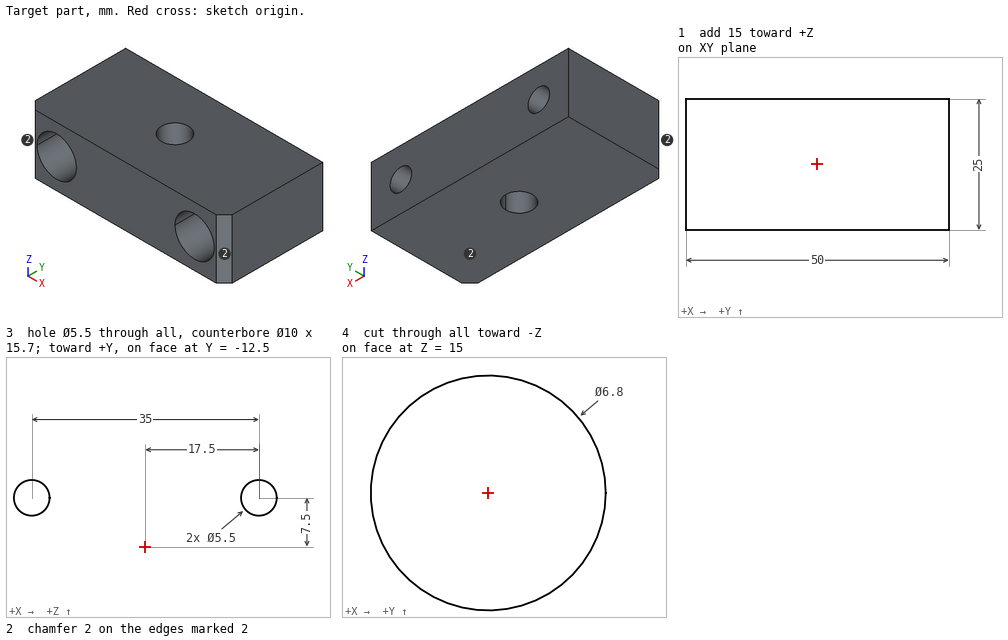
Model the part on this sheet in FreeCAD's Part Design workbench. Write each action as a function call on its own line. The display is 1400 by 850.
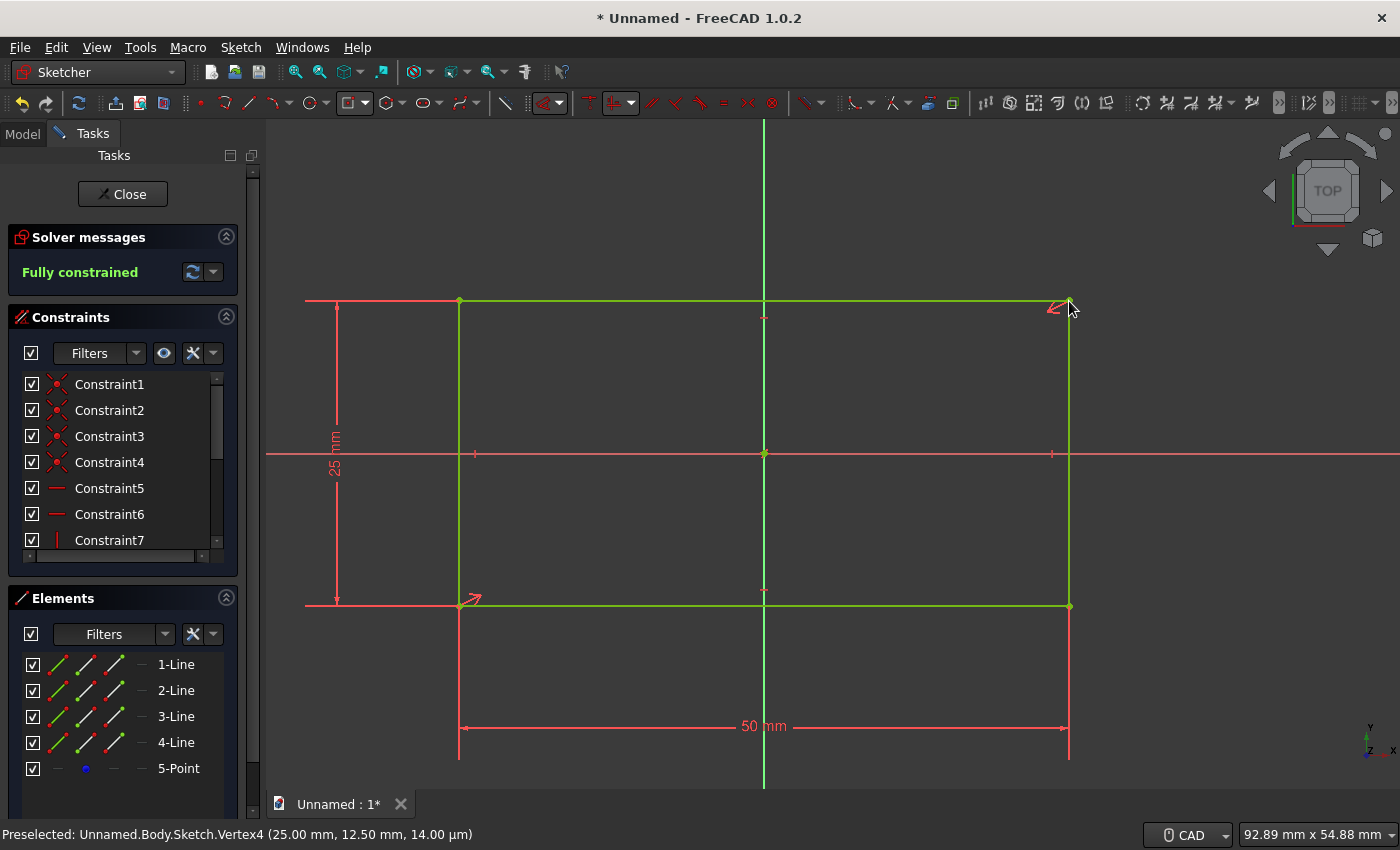
click(123, 194)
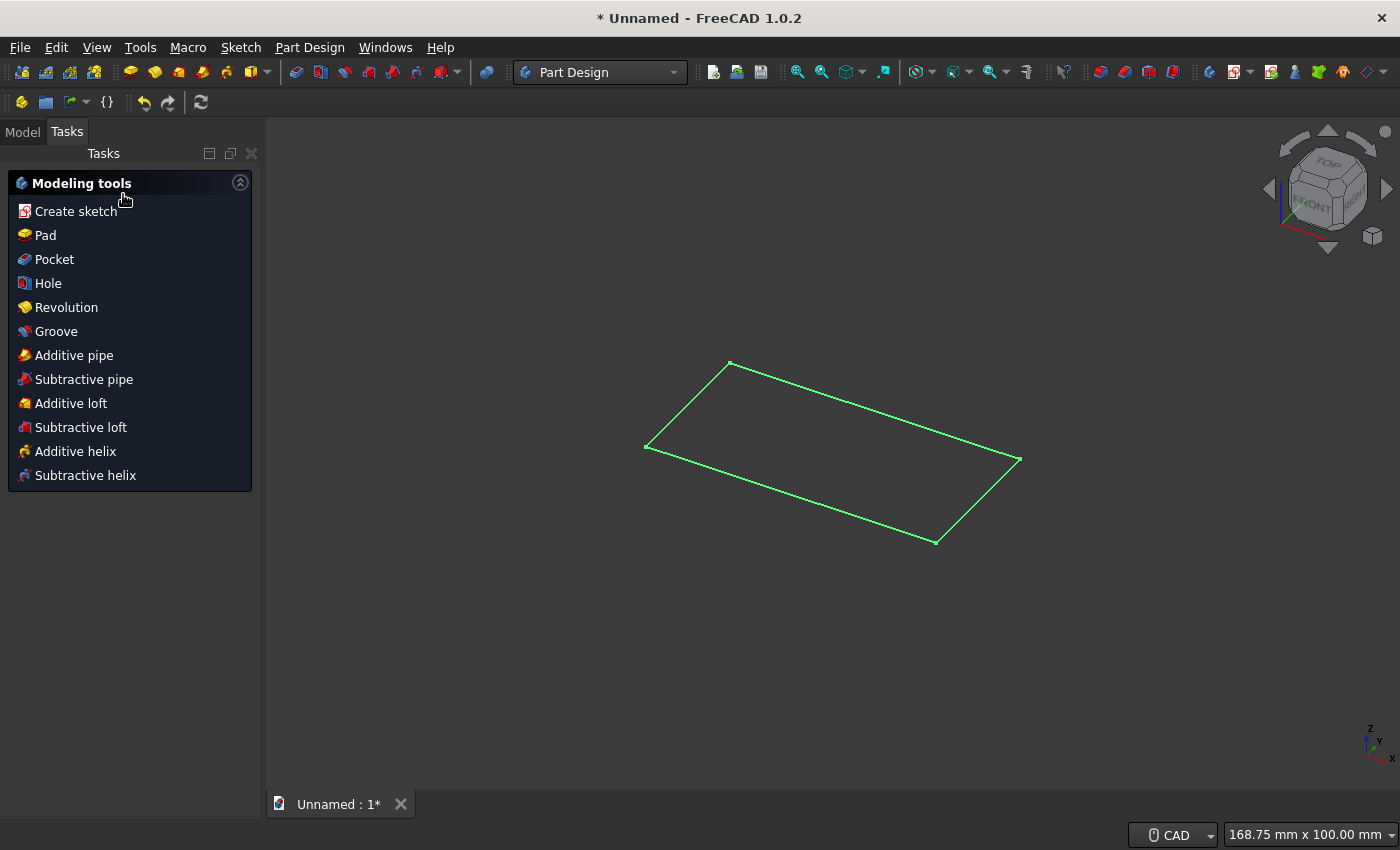
click(132, 72)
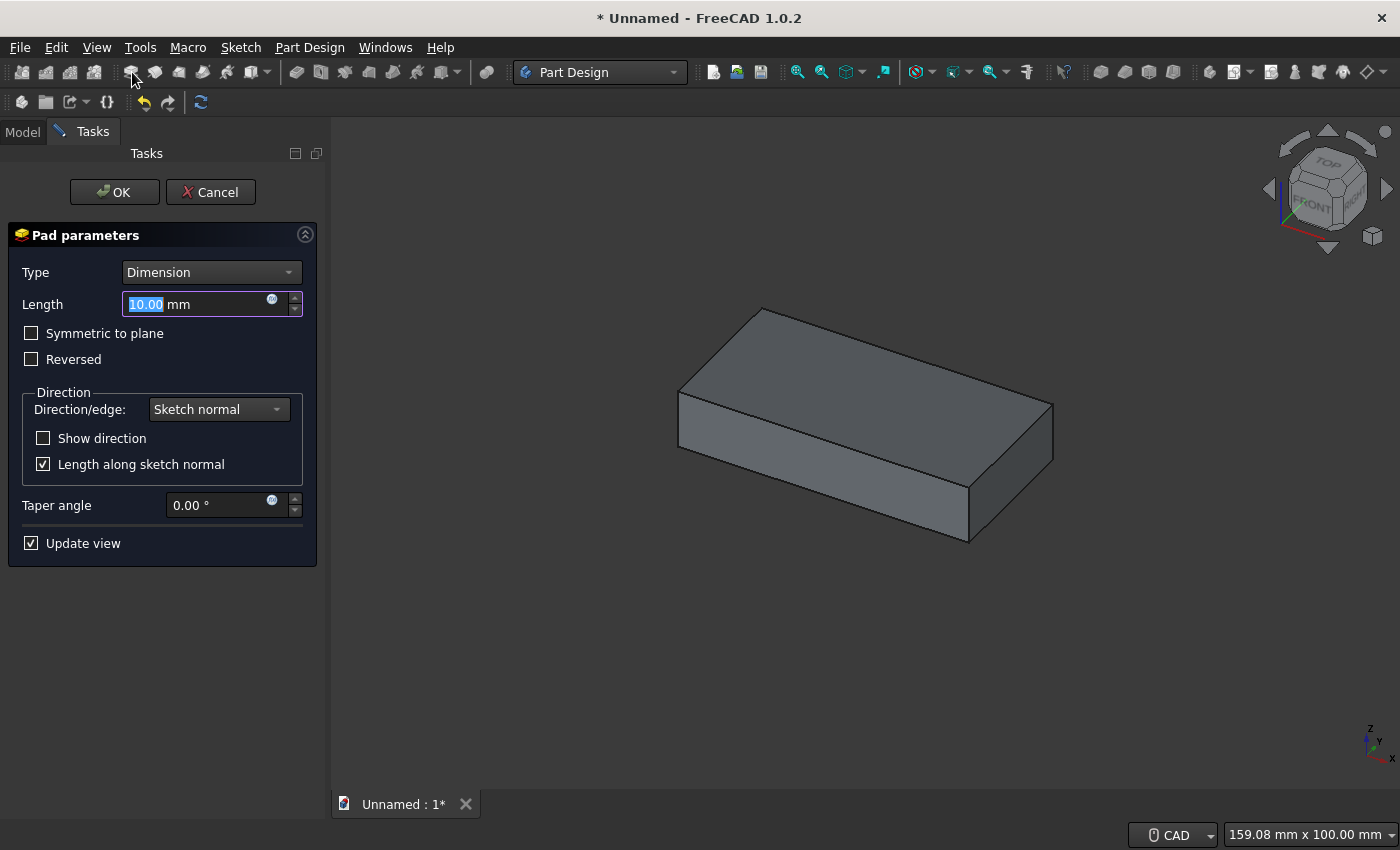
text(15)
key(Tab)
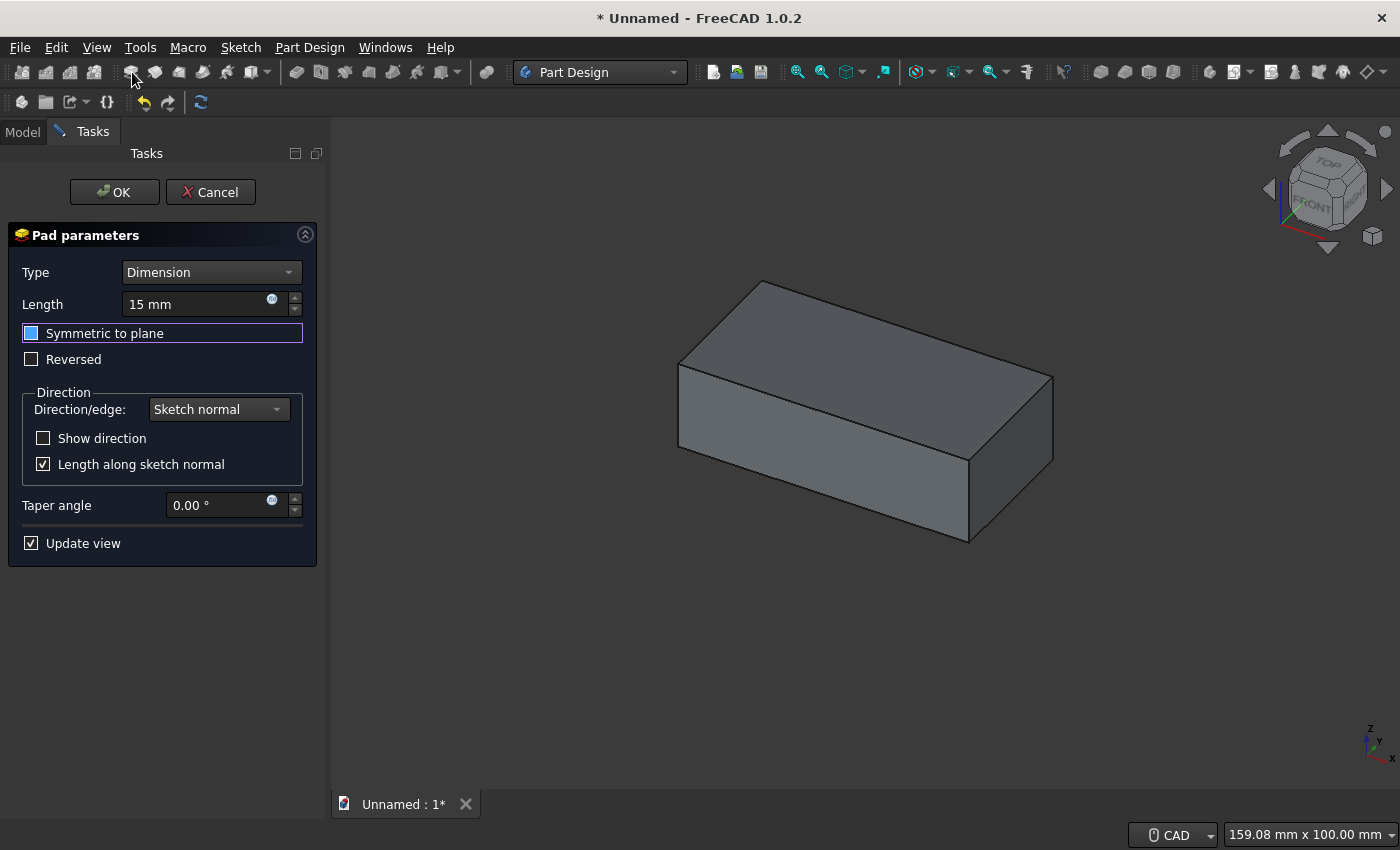
click(115, 192)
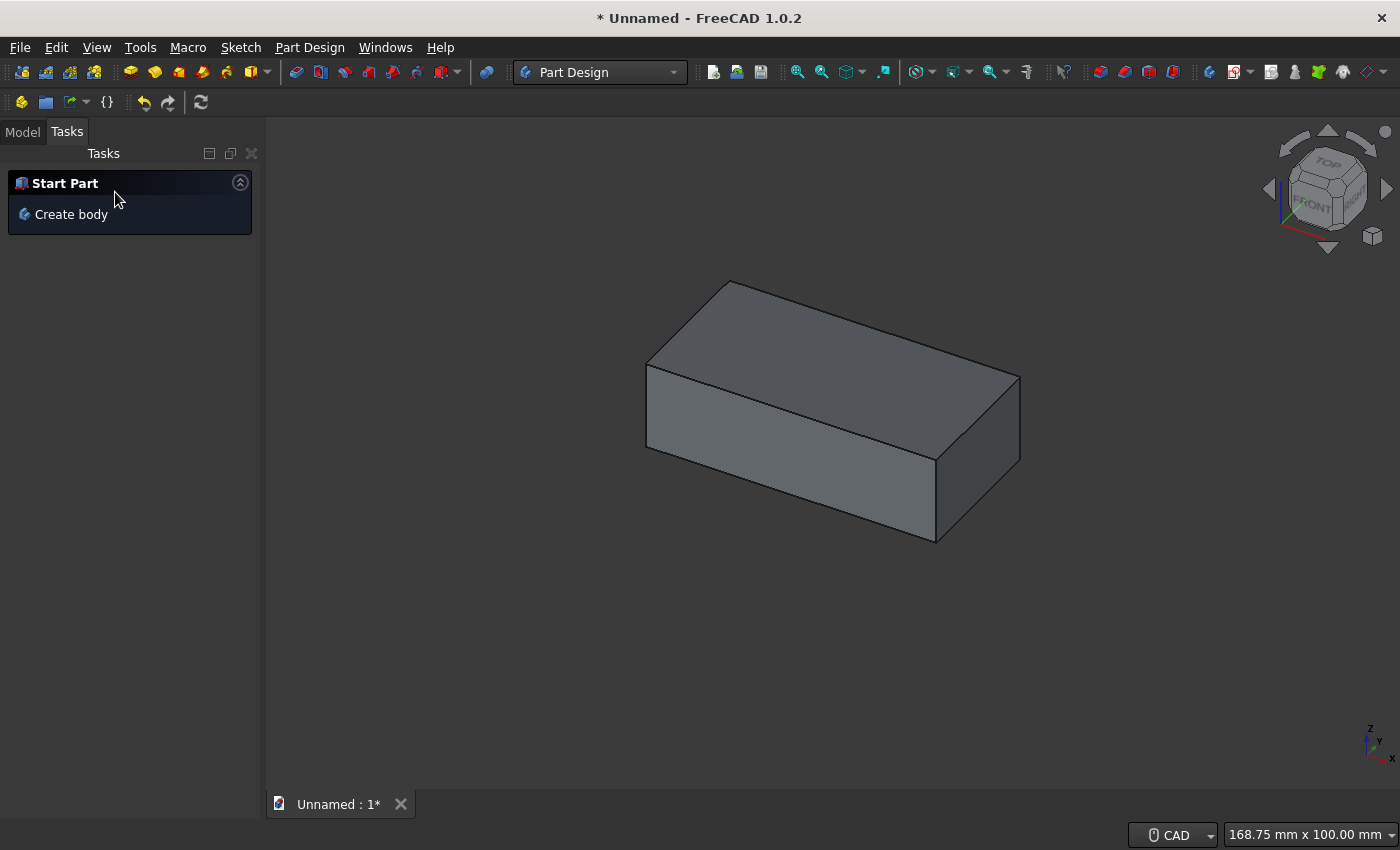
key(v)
key(f)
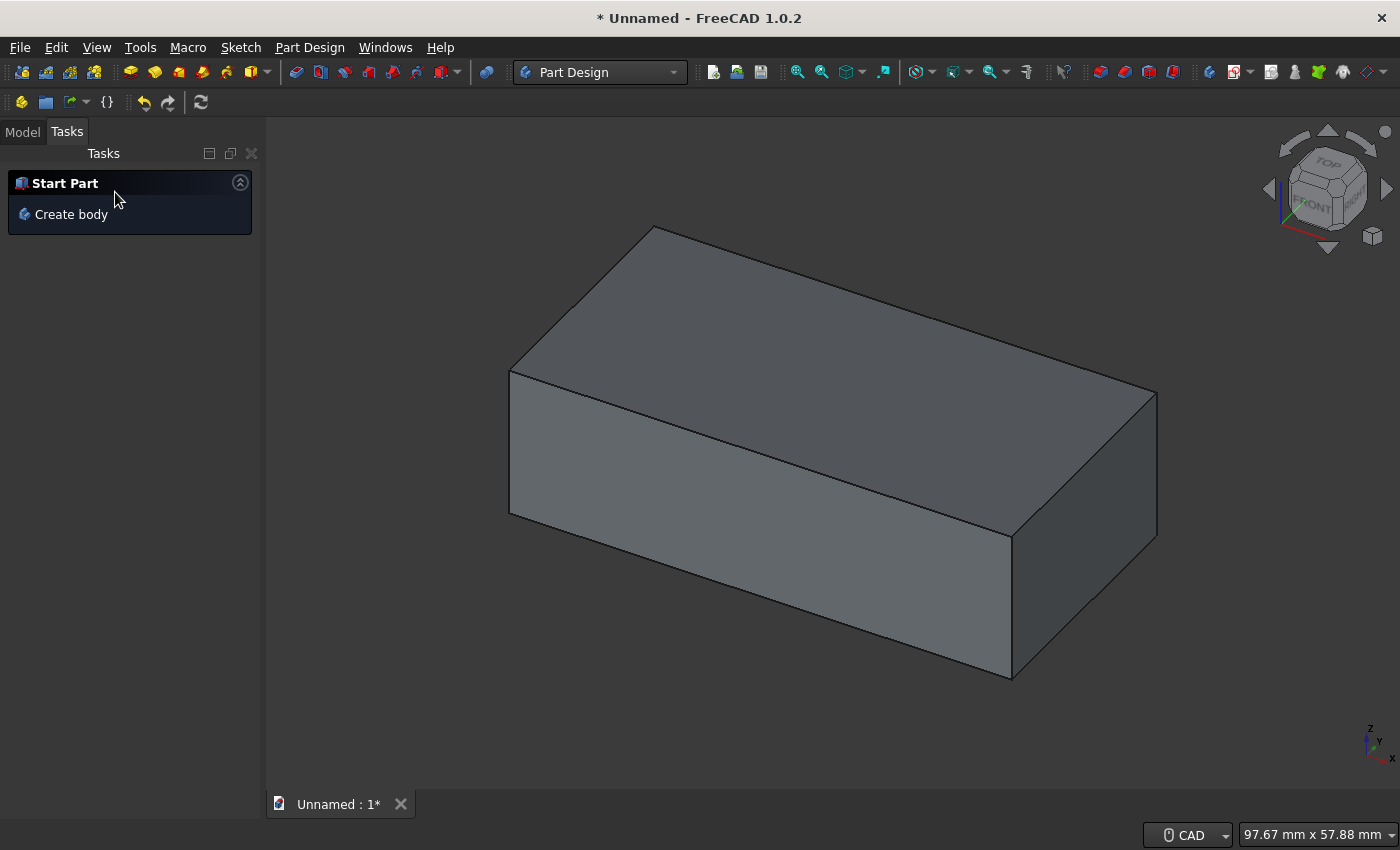
click(1012, 607)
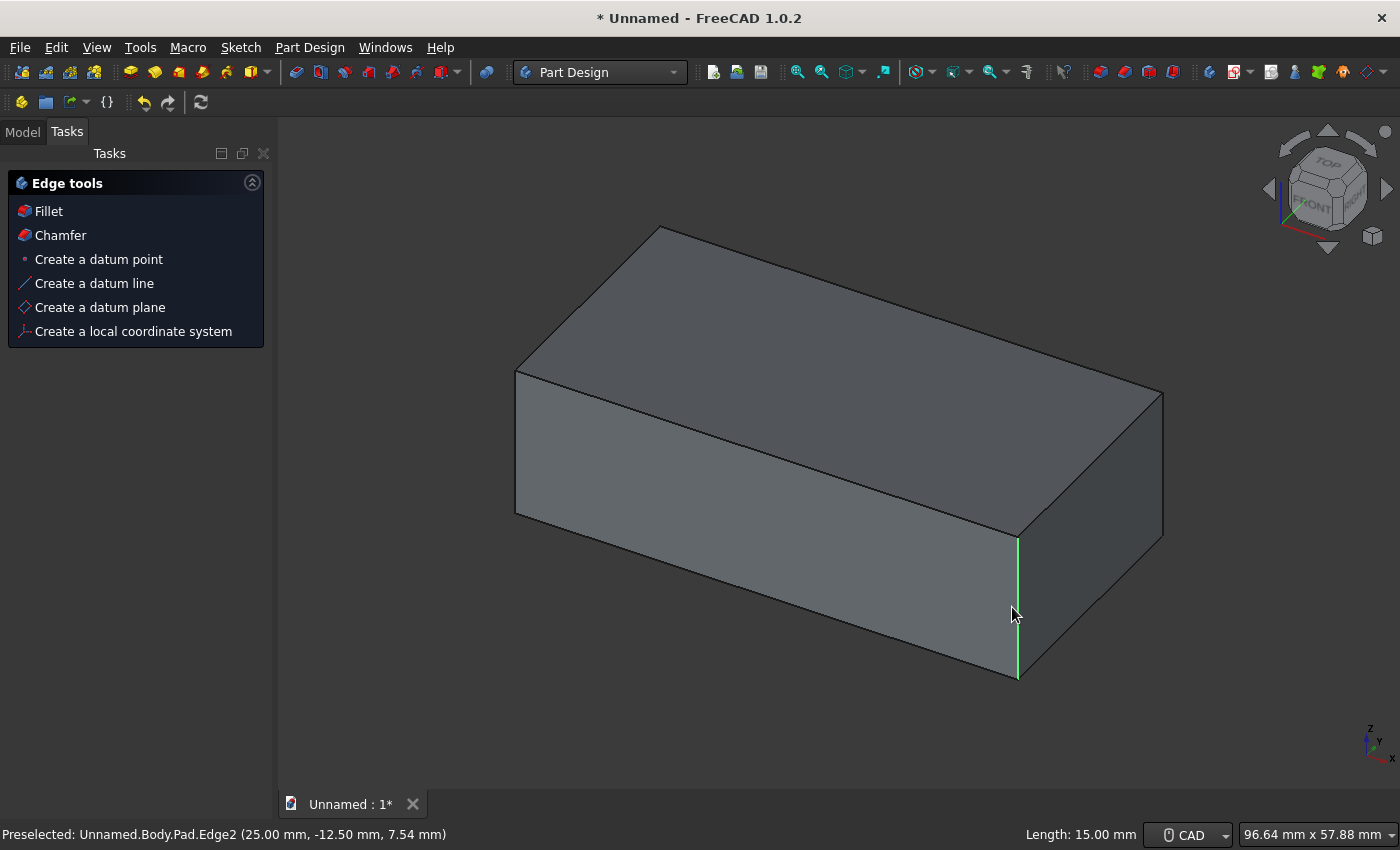
key(0)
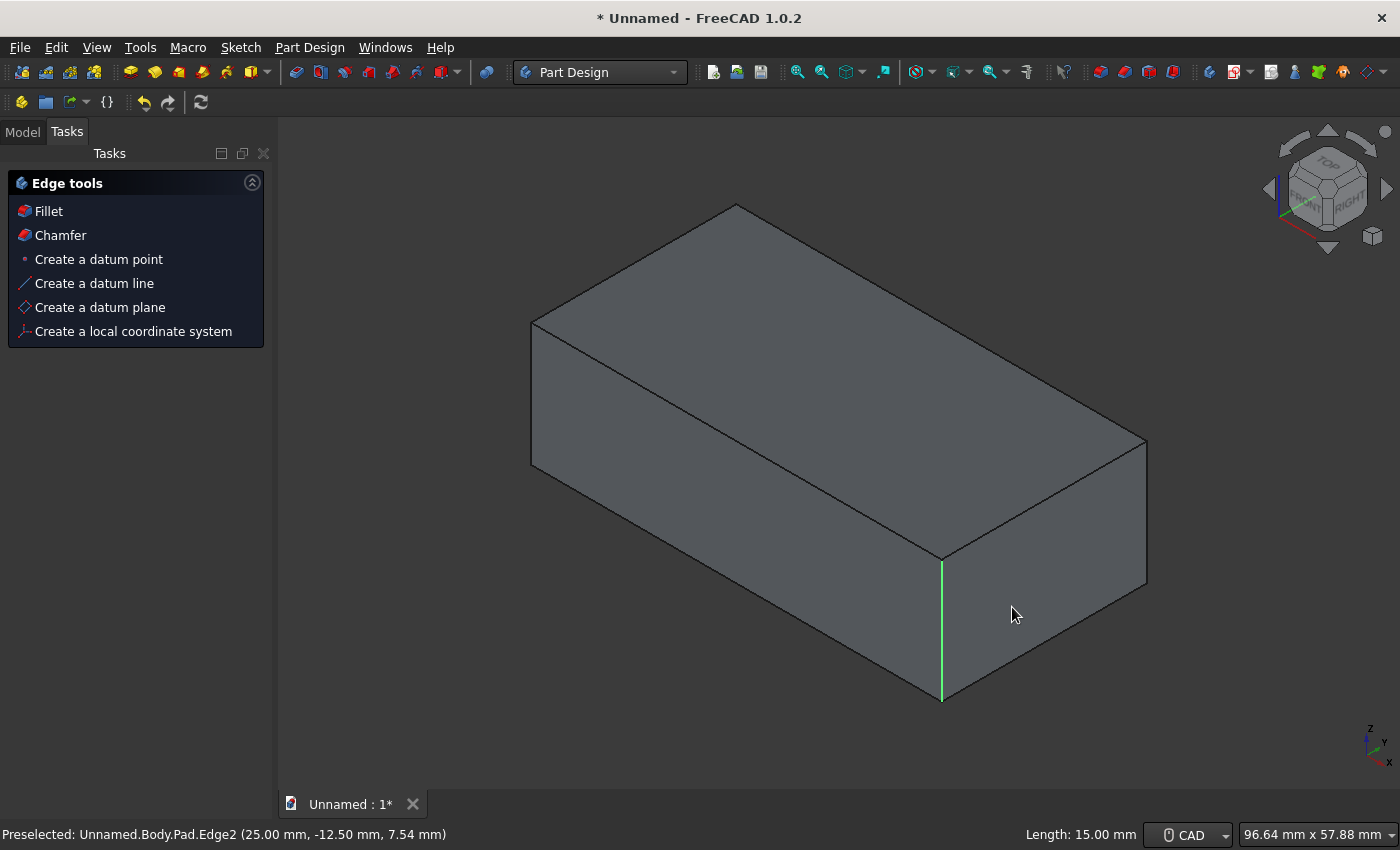
key(2)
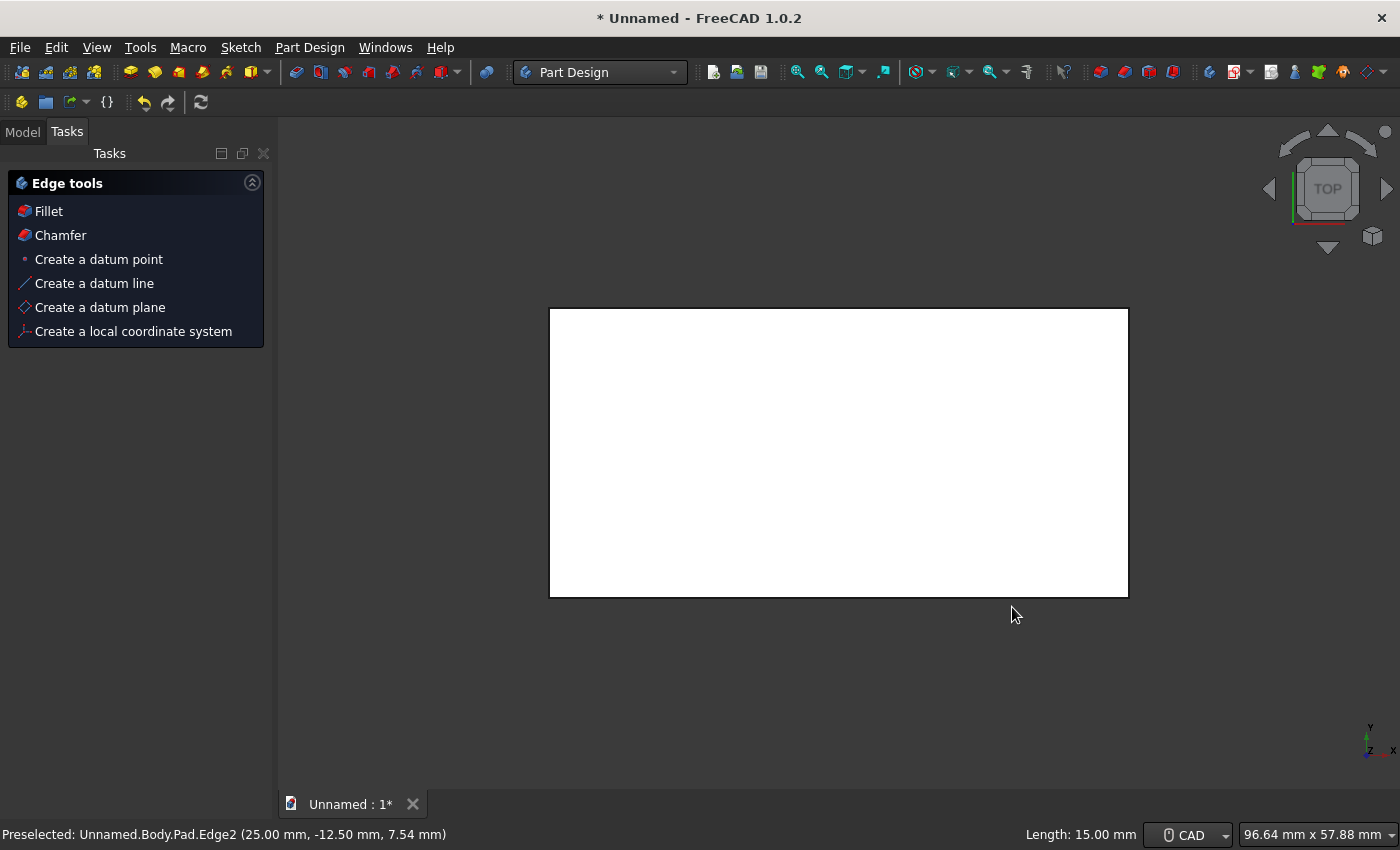
key(1)